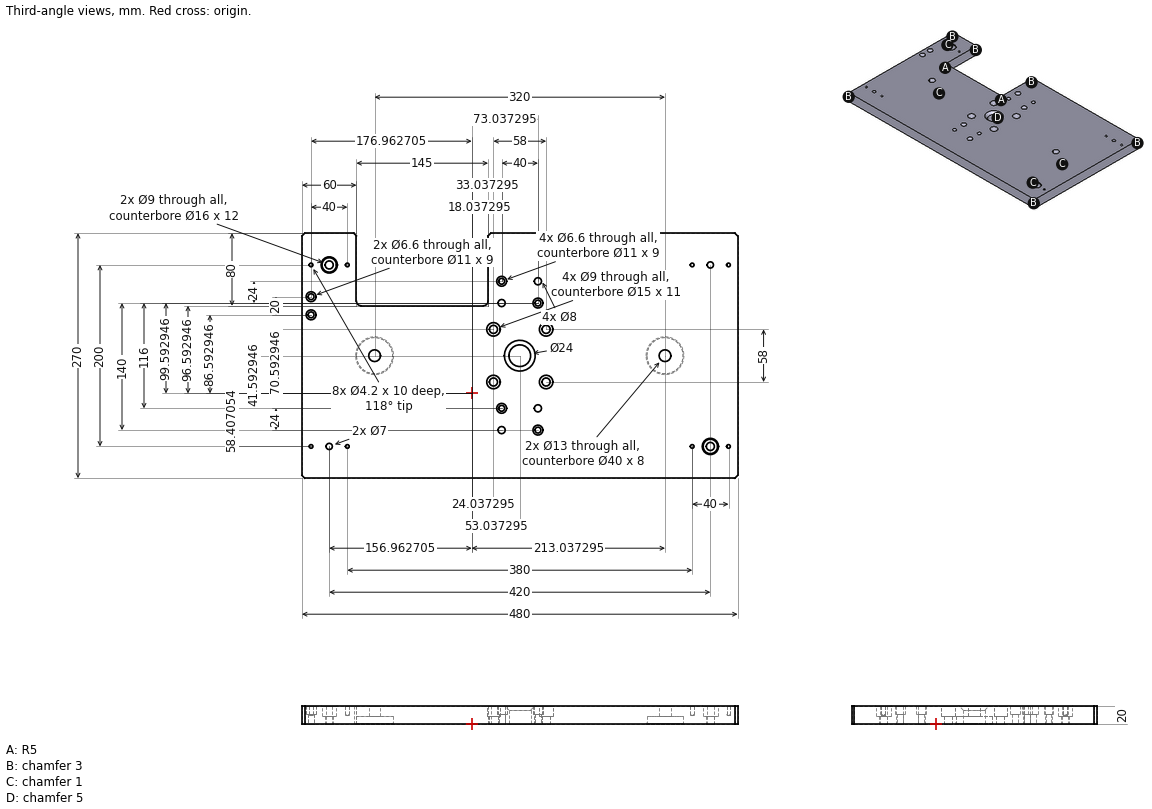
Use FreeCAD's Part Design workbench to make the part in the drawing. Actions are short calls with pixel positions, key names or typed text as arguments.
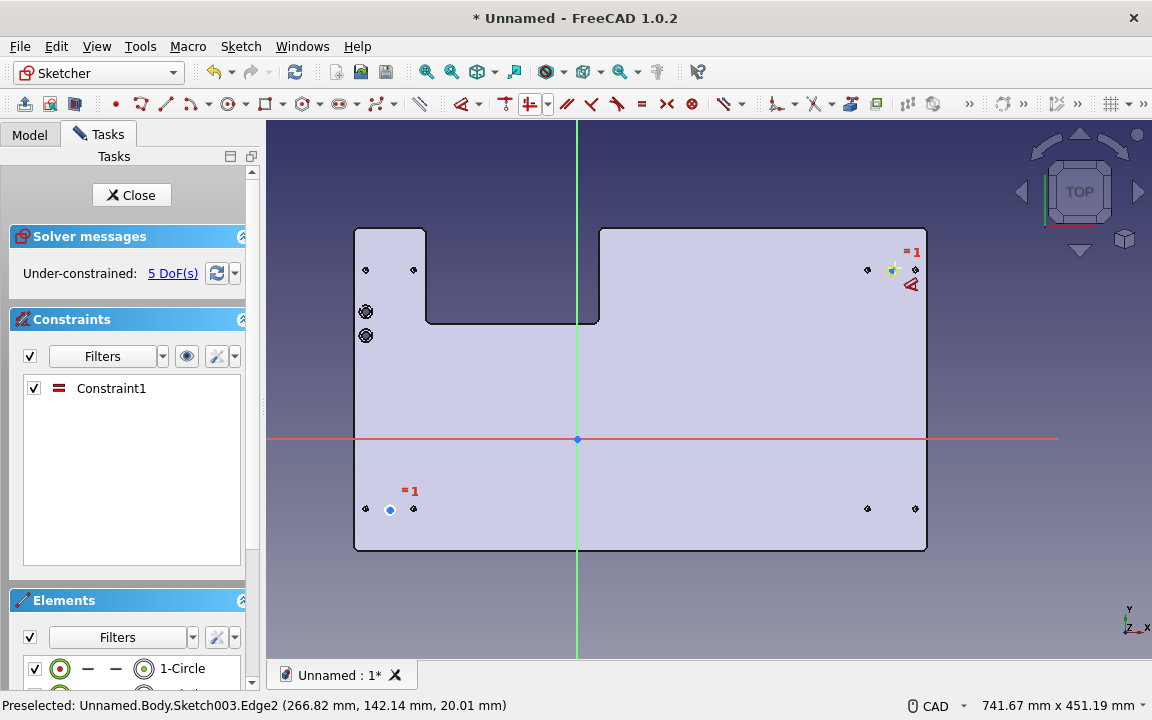
scroll(393, 507, up, 8)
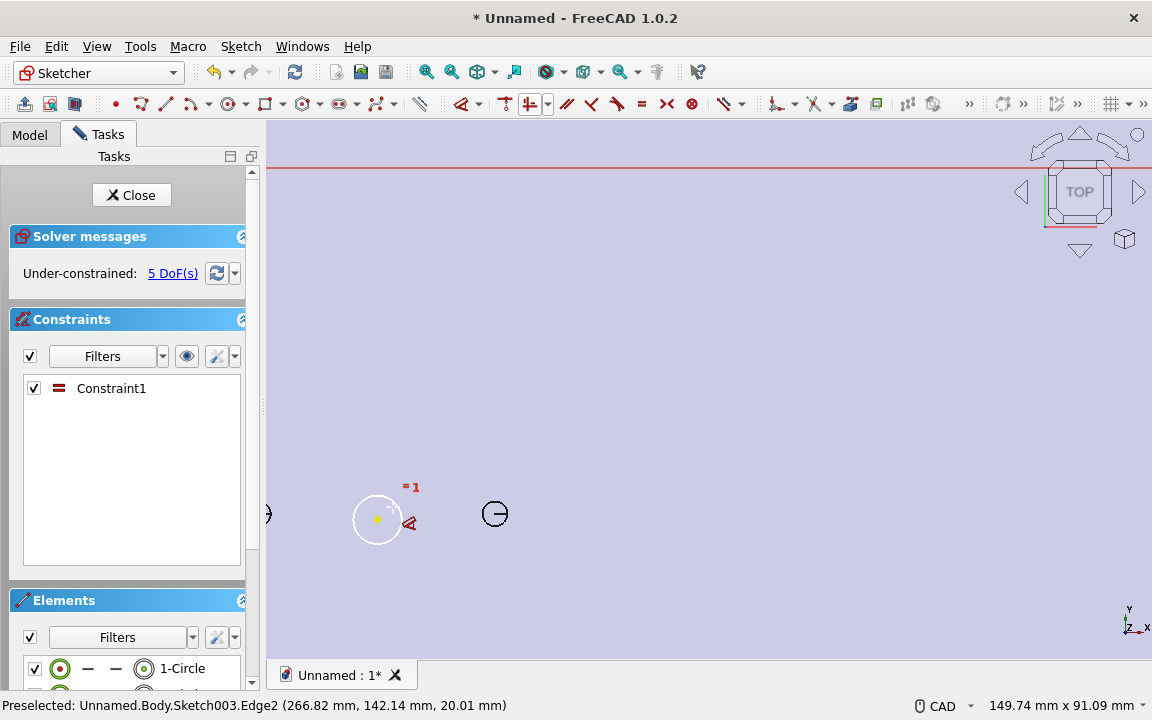
click(395, 503)
click(418, 481)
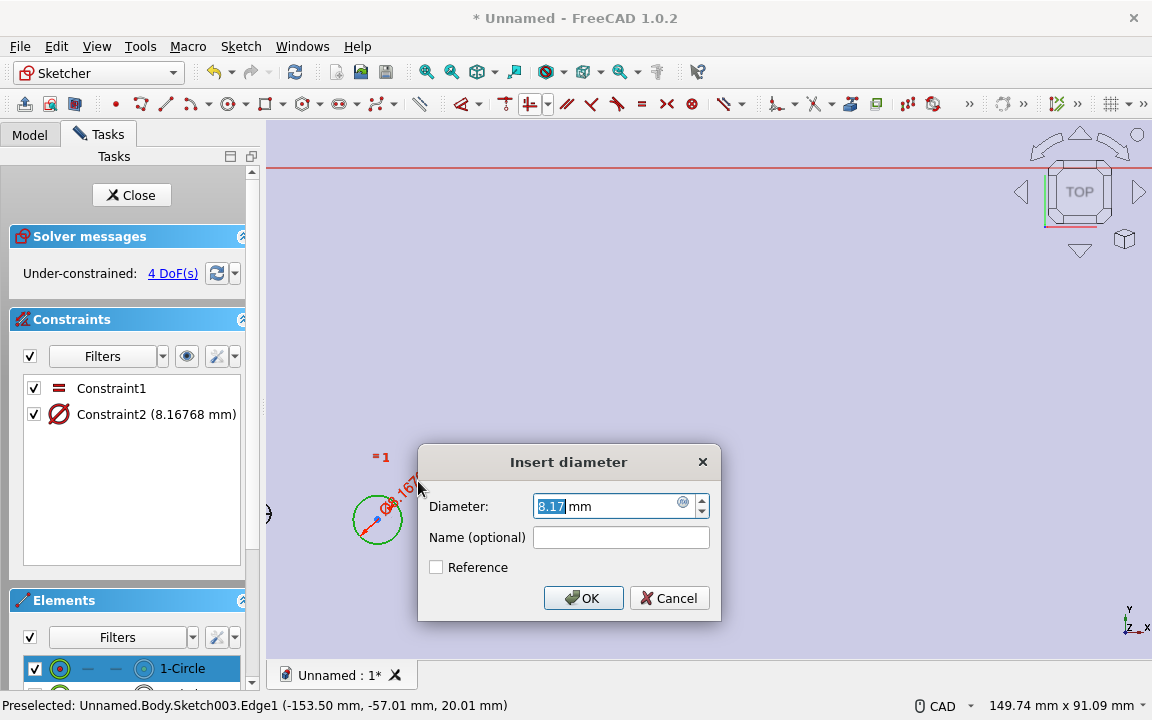
text(7)
key(Return)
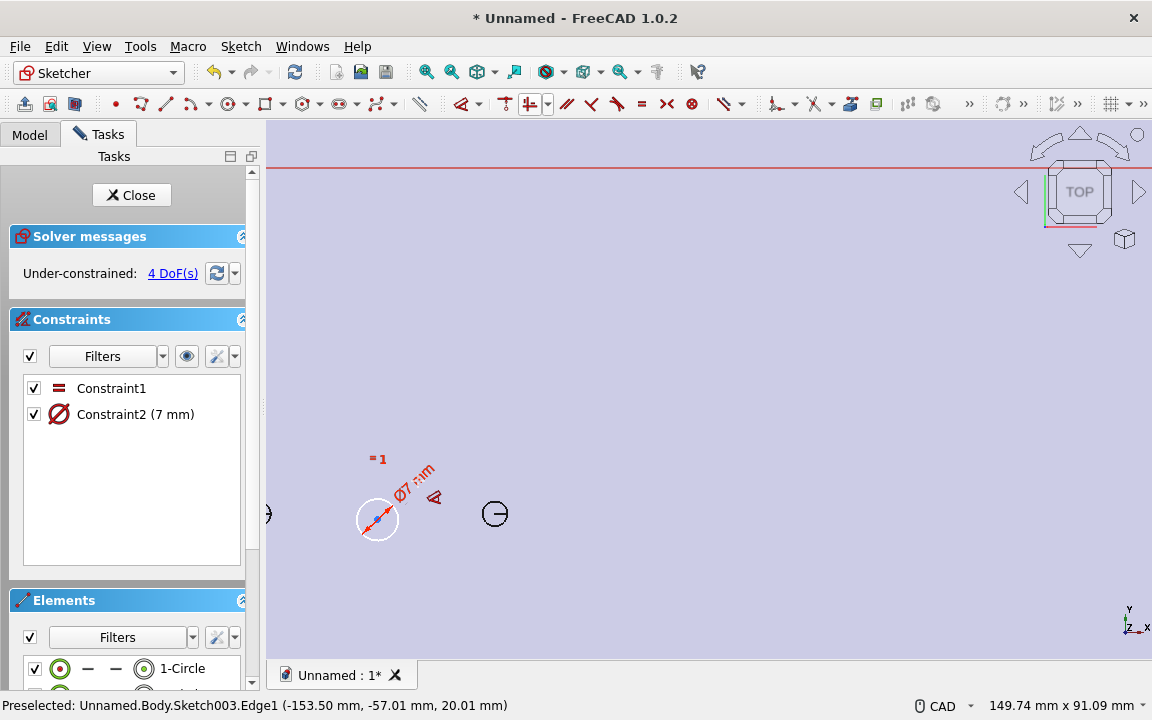
scroll(393, 508, down, 8)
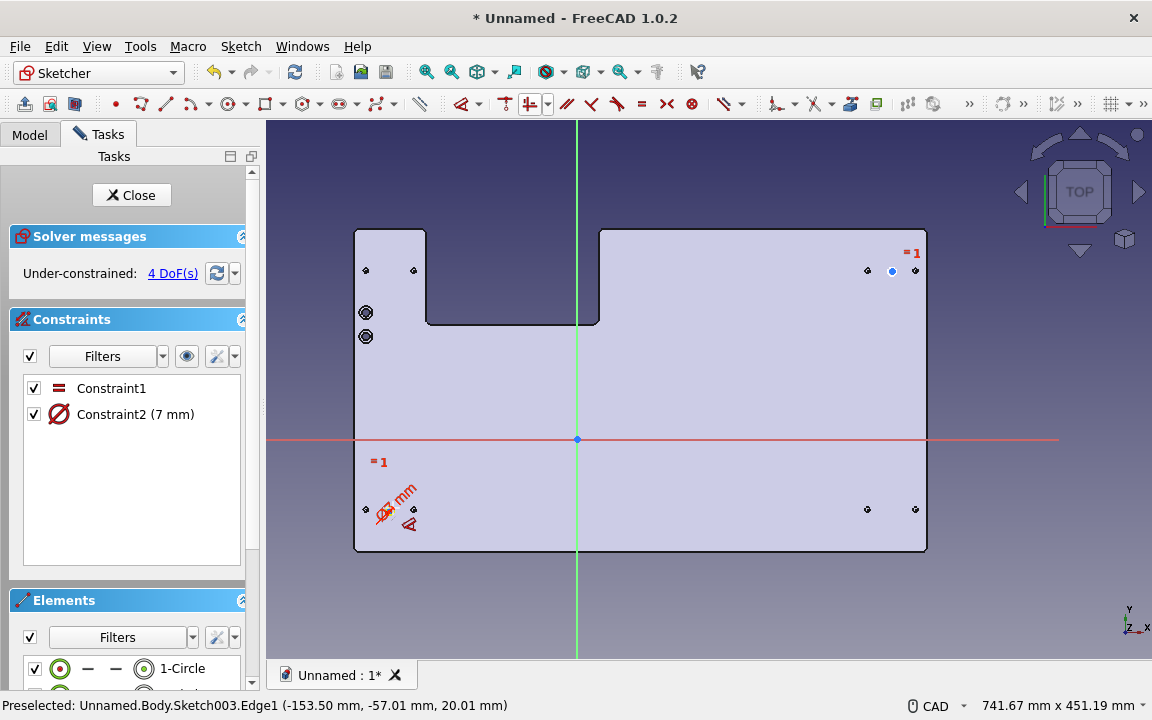
click(390, 511)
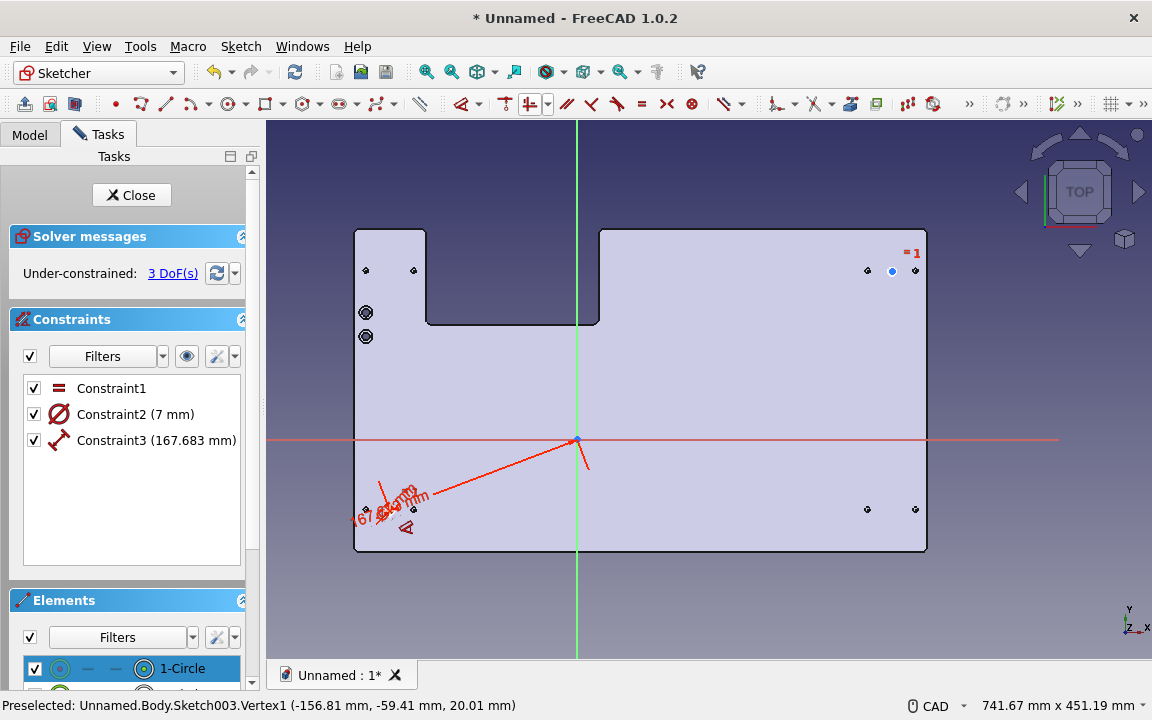
click(892, 272)
click(641, 545)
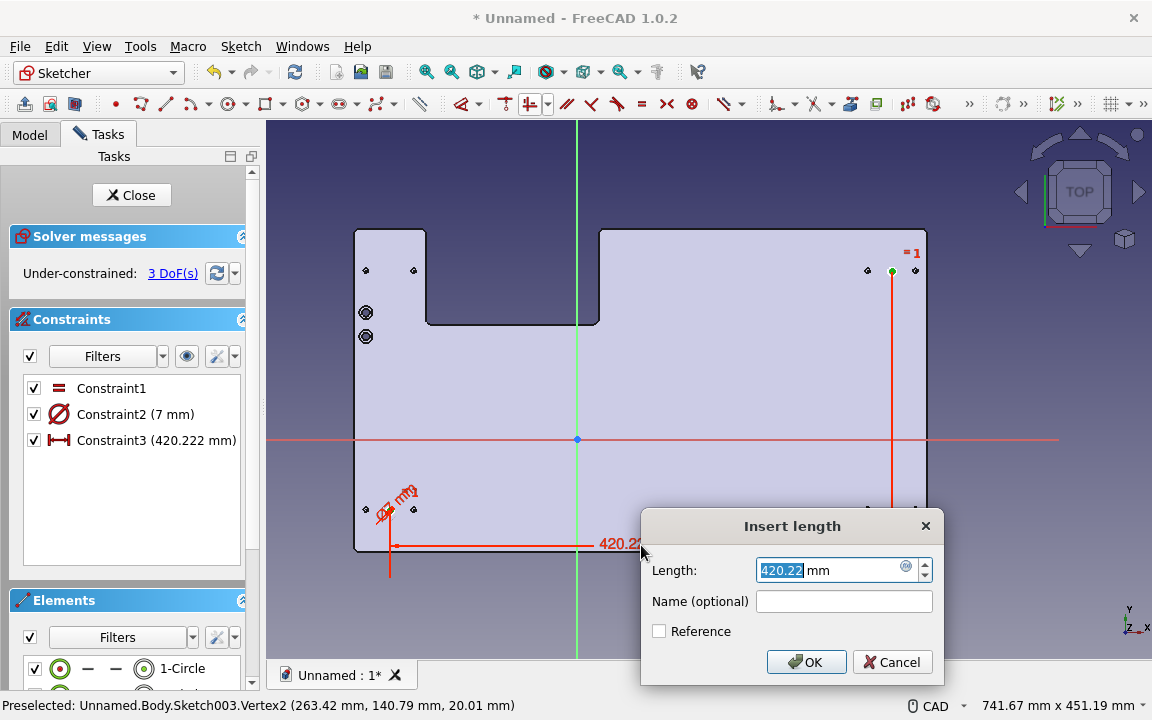
text(420)
key(Return)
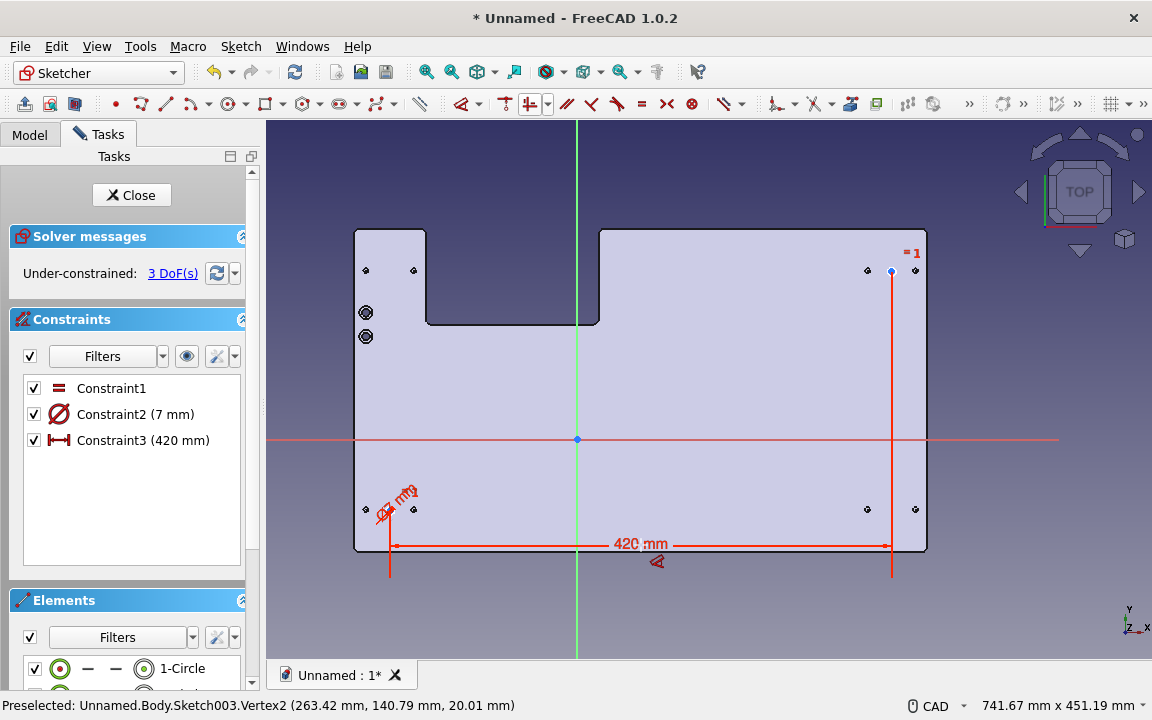
click(390, 511)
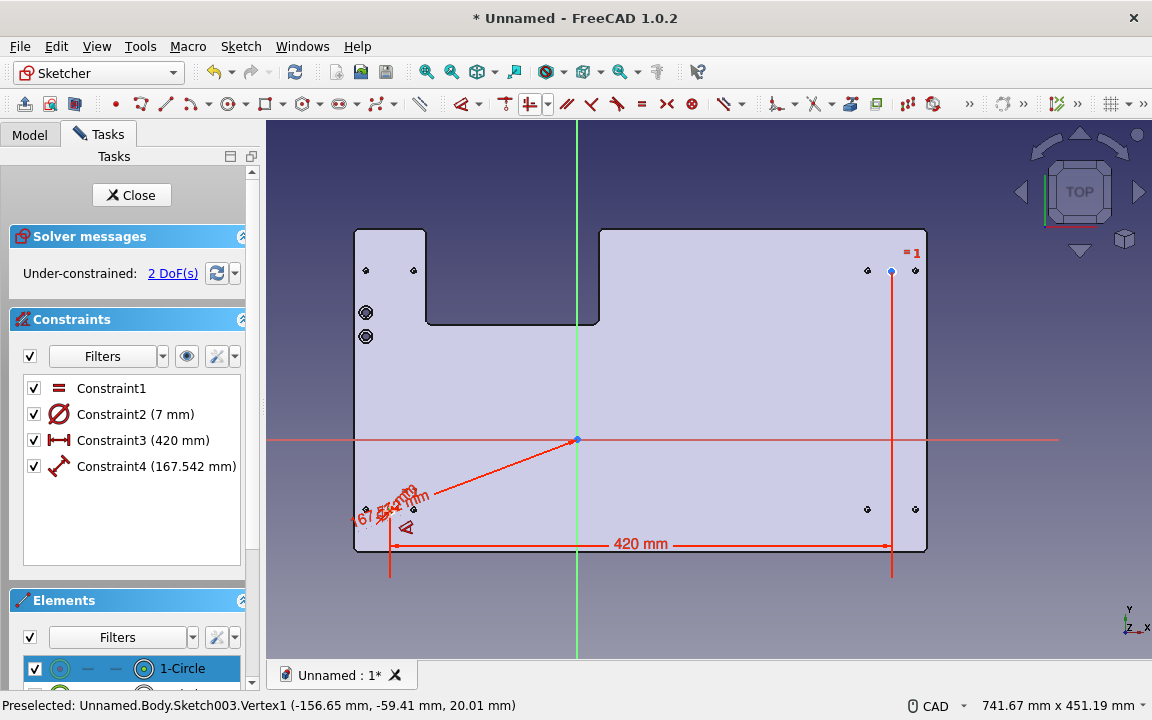
click(892, 272)
click(926, 391)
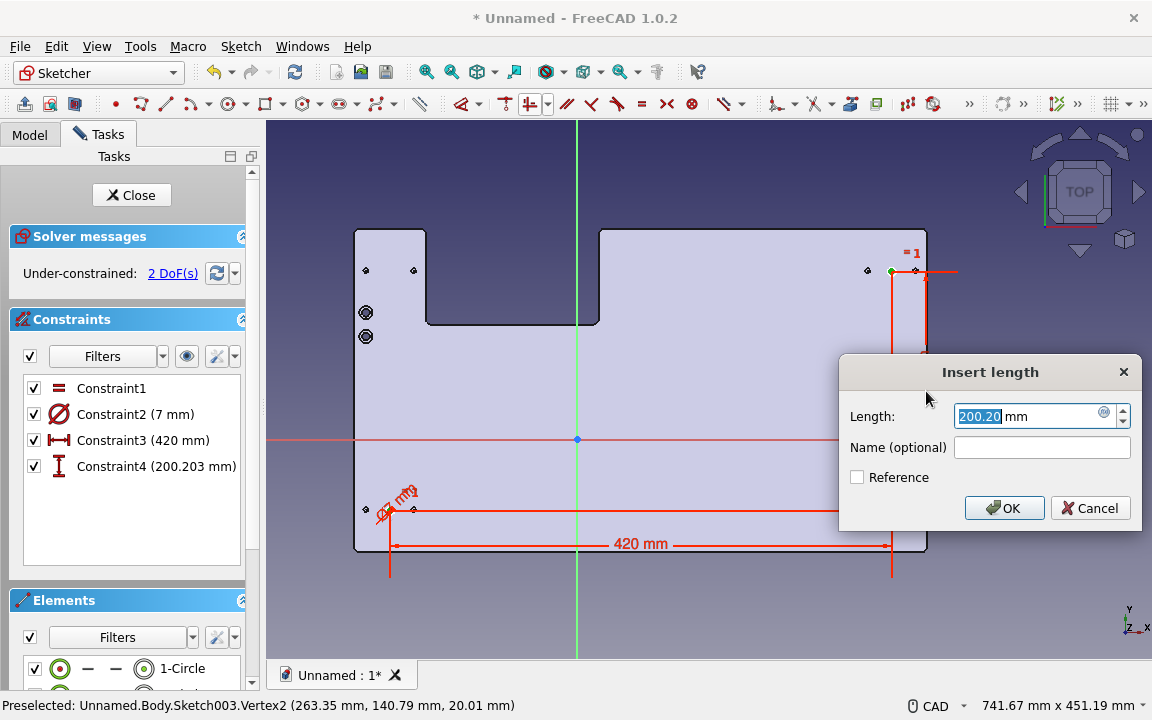
text(200)
key(Return)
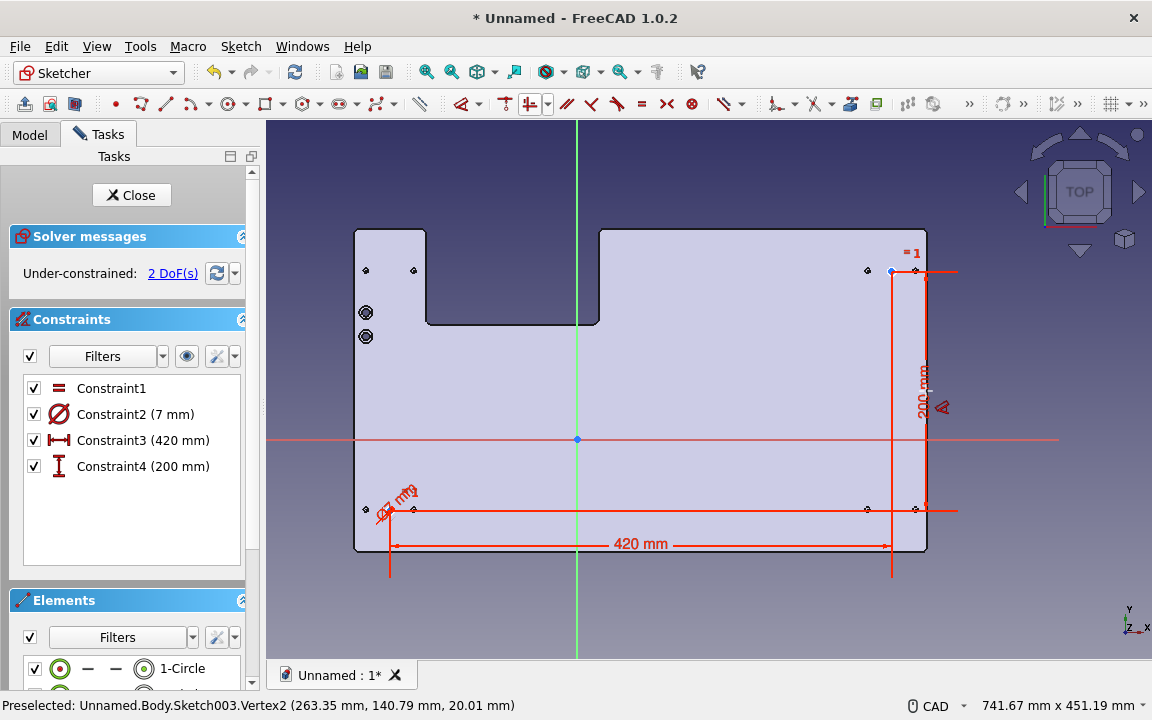
click(390, 511)
click(356, 475)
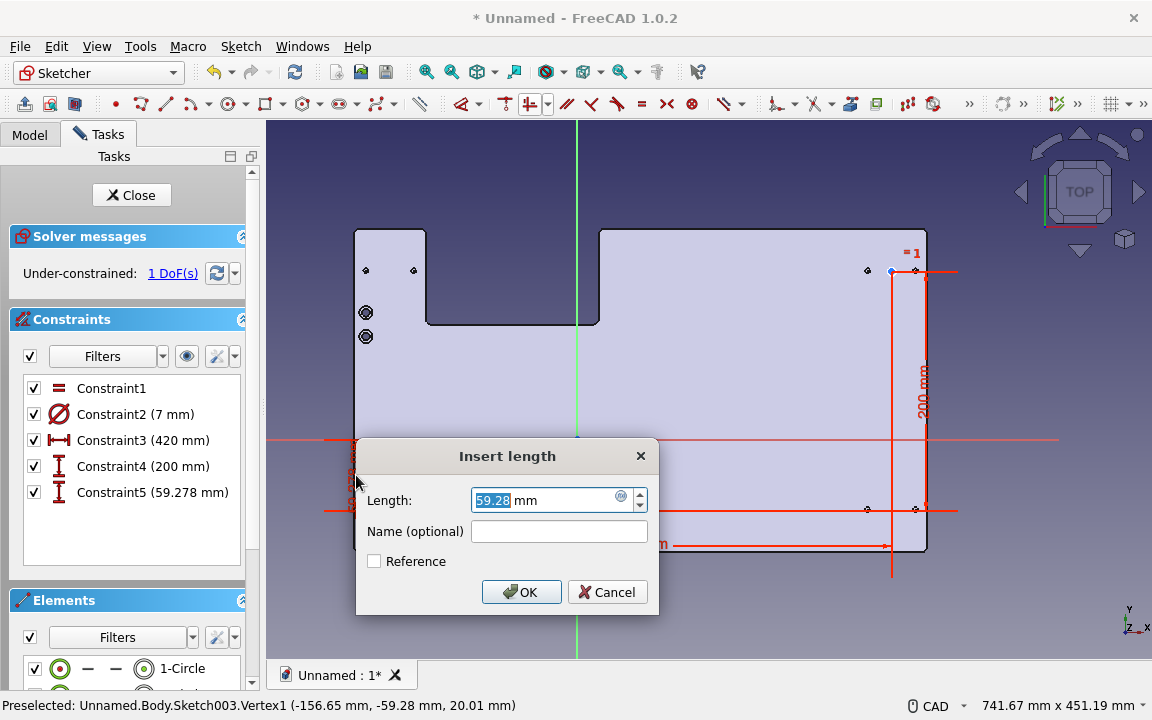
text(58.407054)
key(Return)